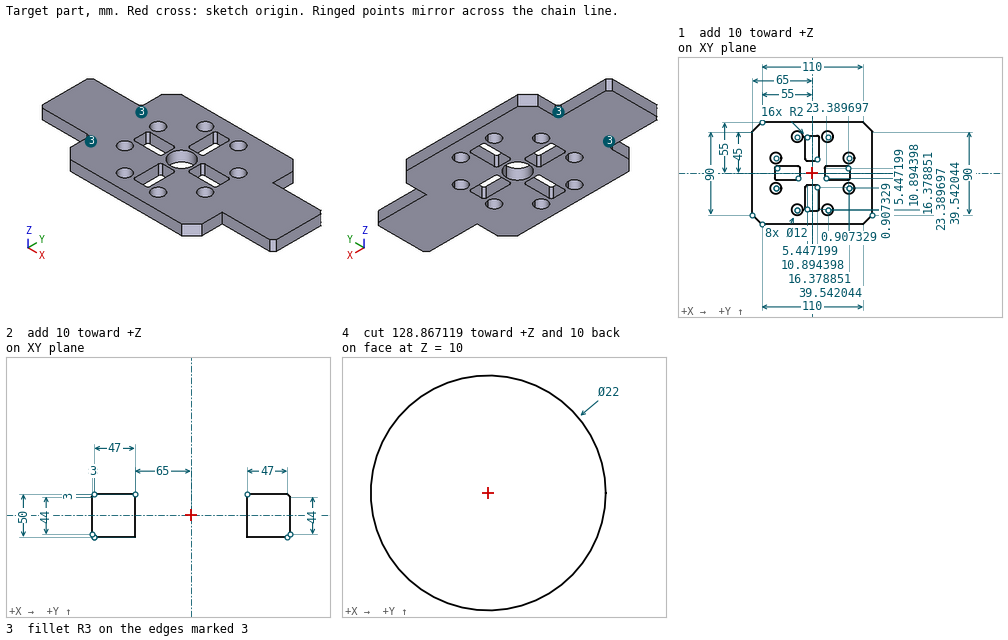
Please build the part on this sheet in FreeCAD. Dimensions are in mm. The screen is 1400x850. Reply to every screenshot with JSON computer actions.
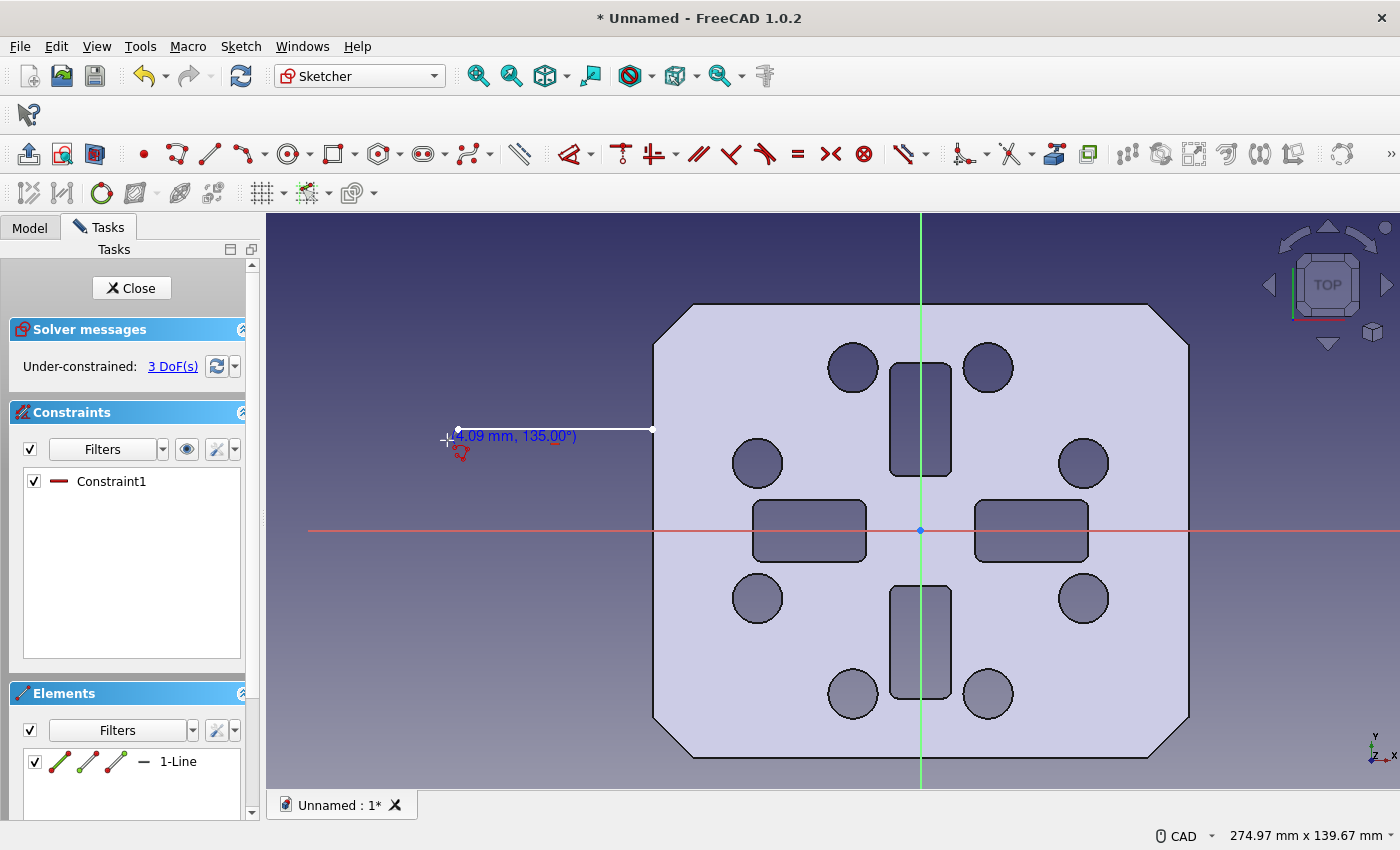
{"action": "left_click", "coordinate": [446, 440]}
{"action": "left_click", "coordinate": [446, 622]}
{"action": "left_click", "coordinate": [459, 634]}
{"action": "left_click", "coordinate": [653, 634]}
{"action": "left_click", "coordinate": [653, 429]}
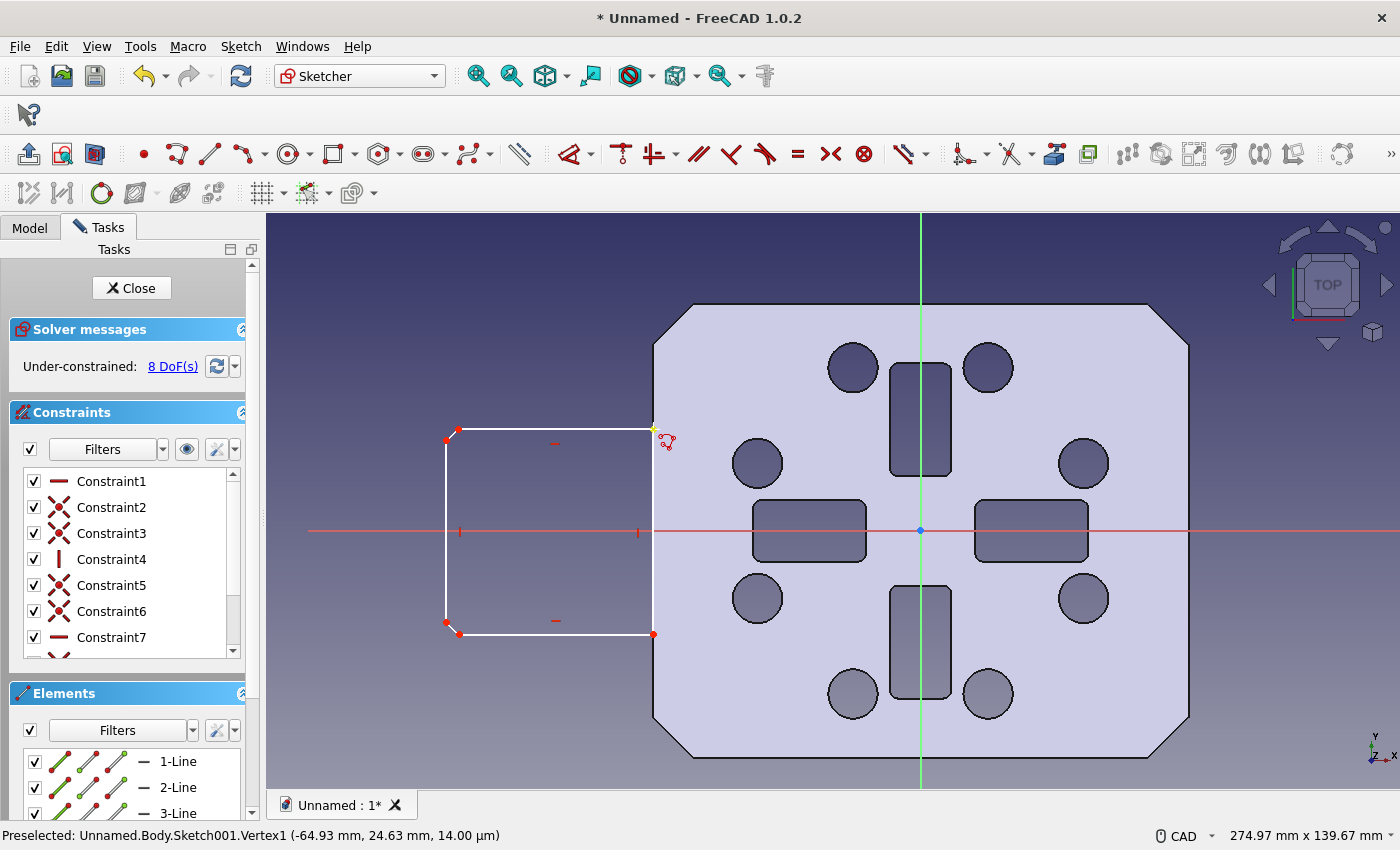
{"action": "left_click", "coordinate": [1189, 428]}
{"action": "left_click", "coordinate": [1189, 634]}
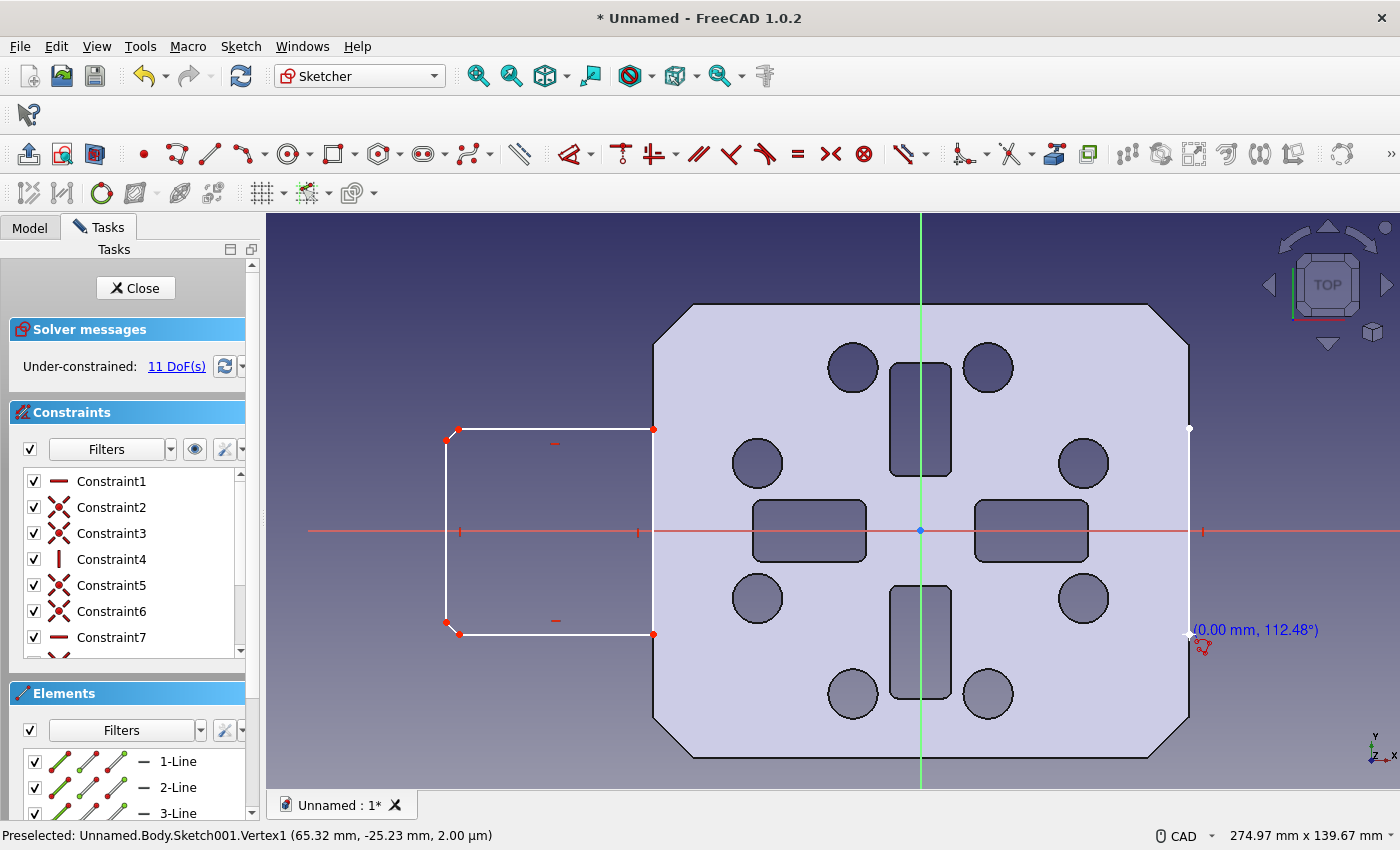
{"action": "scroll", "coordinate": [447, 440], "scroll_direction": "down", "scroll_amount": 2}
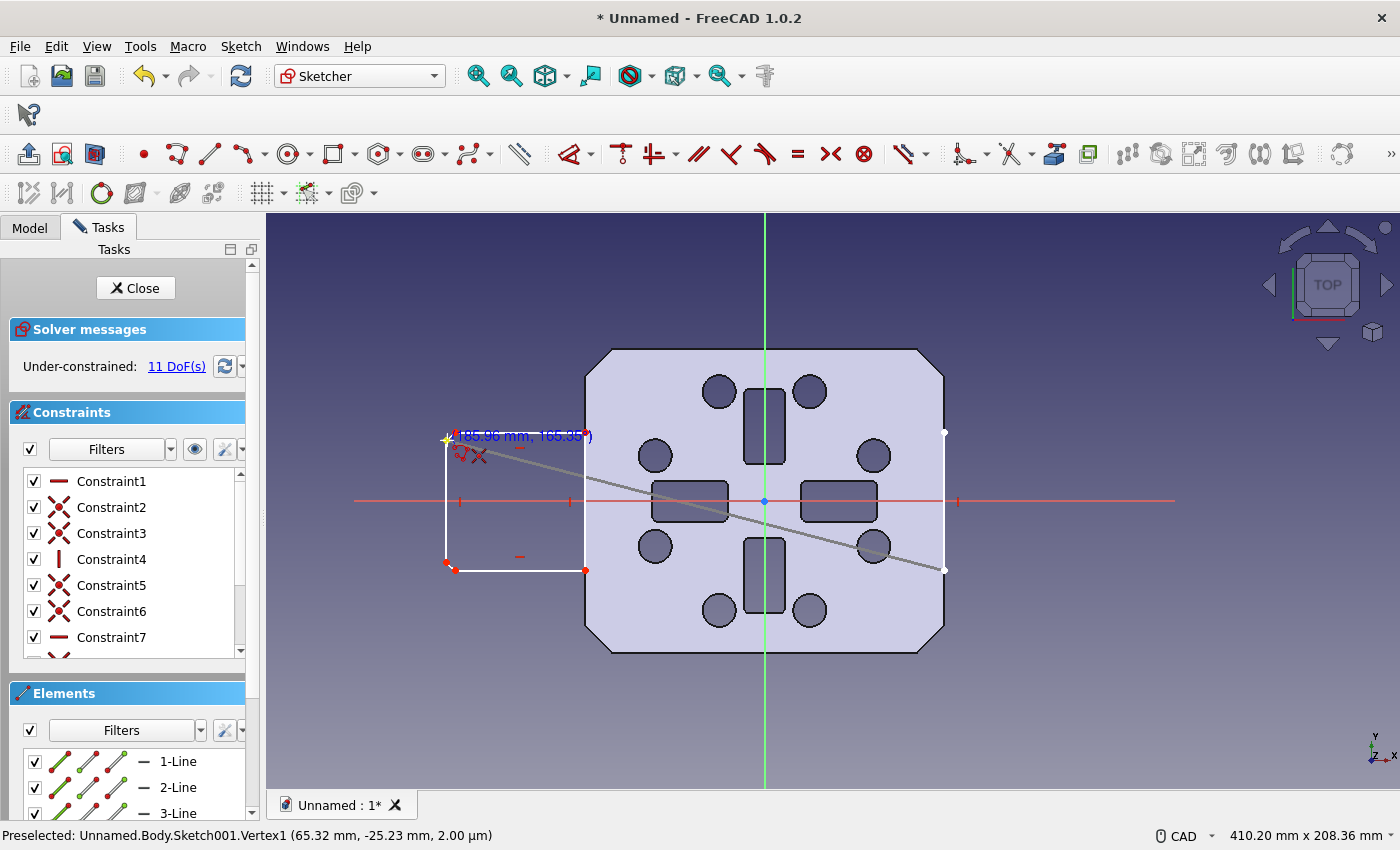
{"action": "left_click", "coordinate": [1074, 570]}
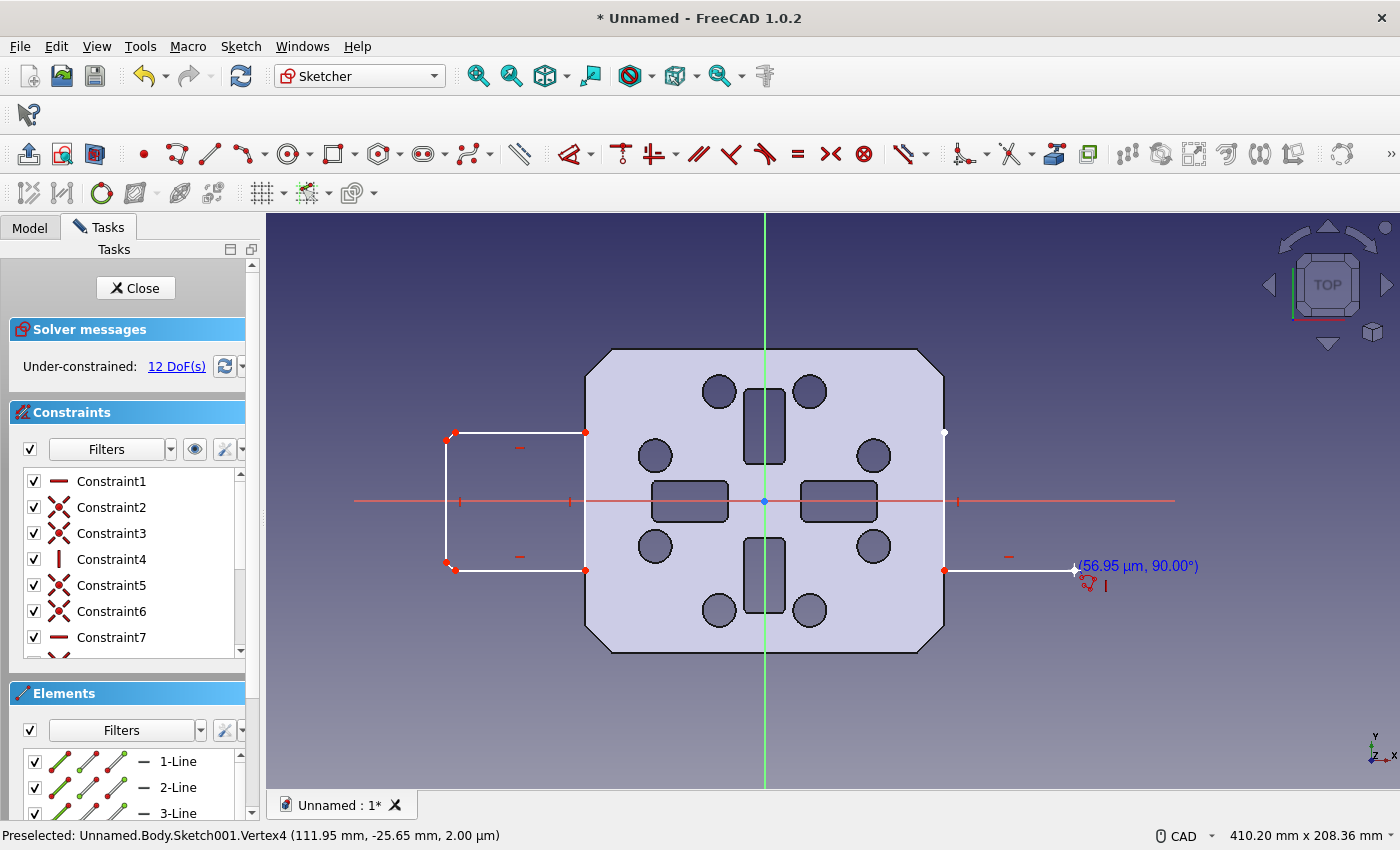
{"action": "scroll", "coordinate": [1082, 562], "scroll_direction": "up", "scroll_amount": 2}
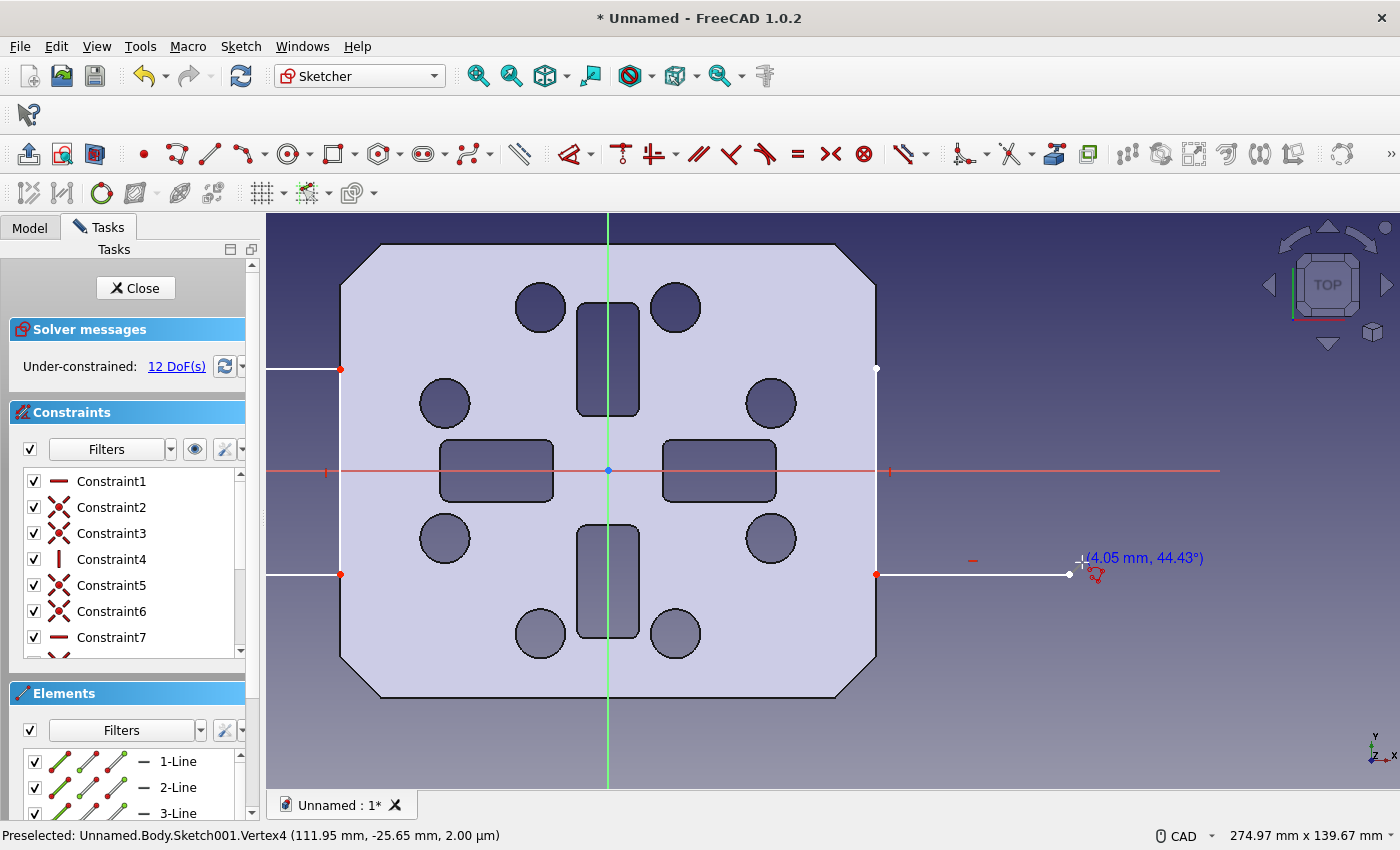
{"action": "left_click", "coordinate": [1082, 562]}
{"action": "left_click", "coordinate": [1082, 380]}
{"action": "left_click", "coordinate": [1070, 368]}
{"action": "left_click", "coordinate": [876, 369]}
{"action": "key", "text": "Escape"}
{"action": "key", "text": "Escape"}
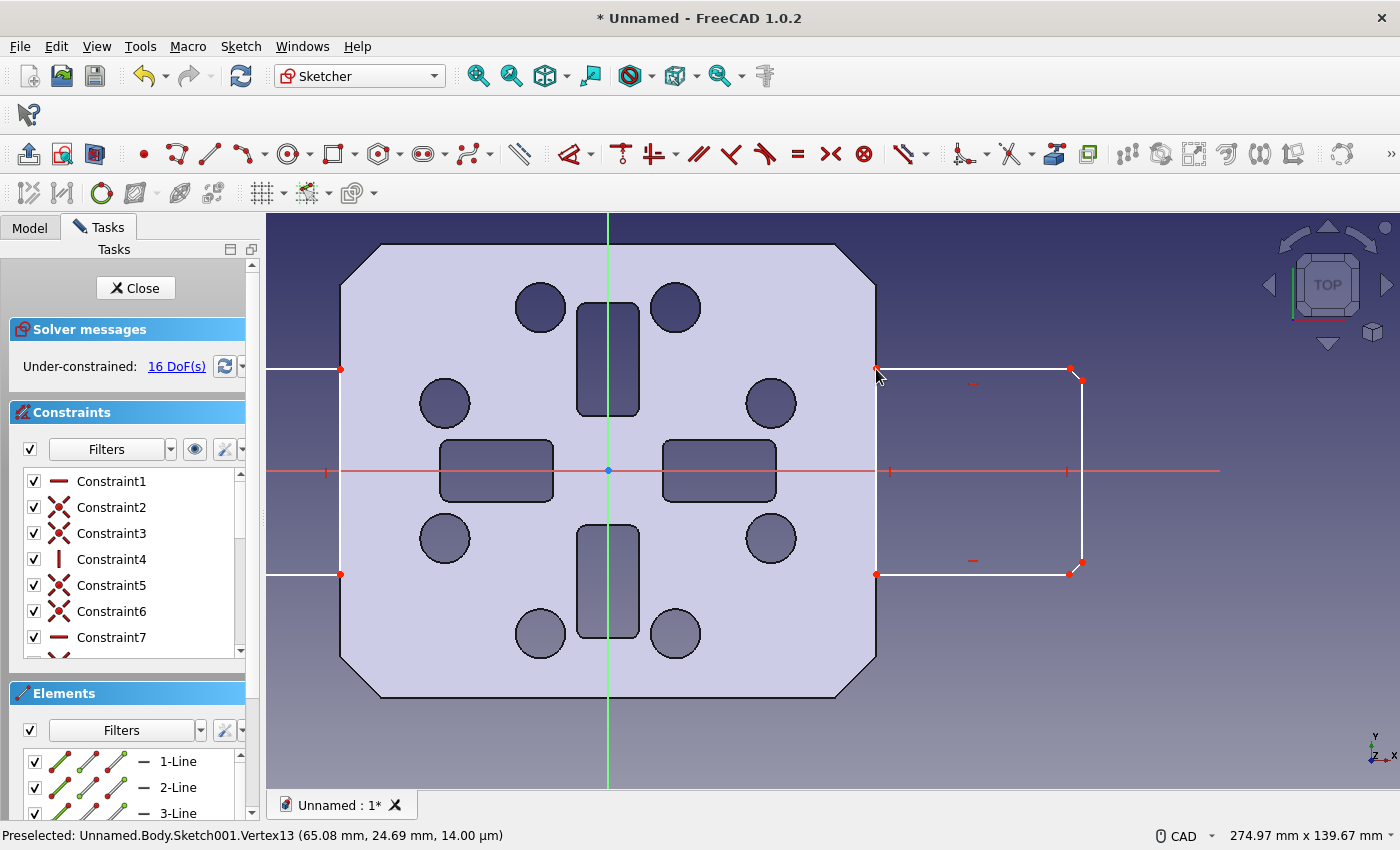
{"action": "scroll", "coordinate": [1083, 562], "scroll_direction": "down", "scroll_amount": 2}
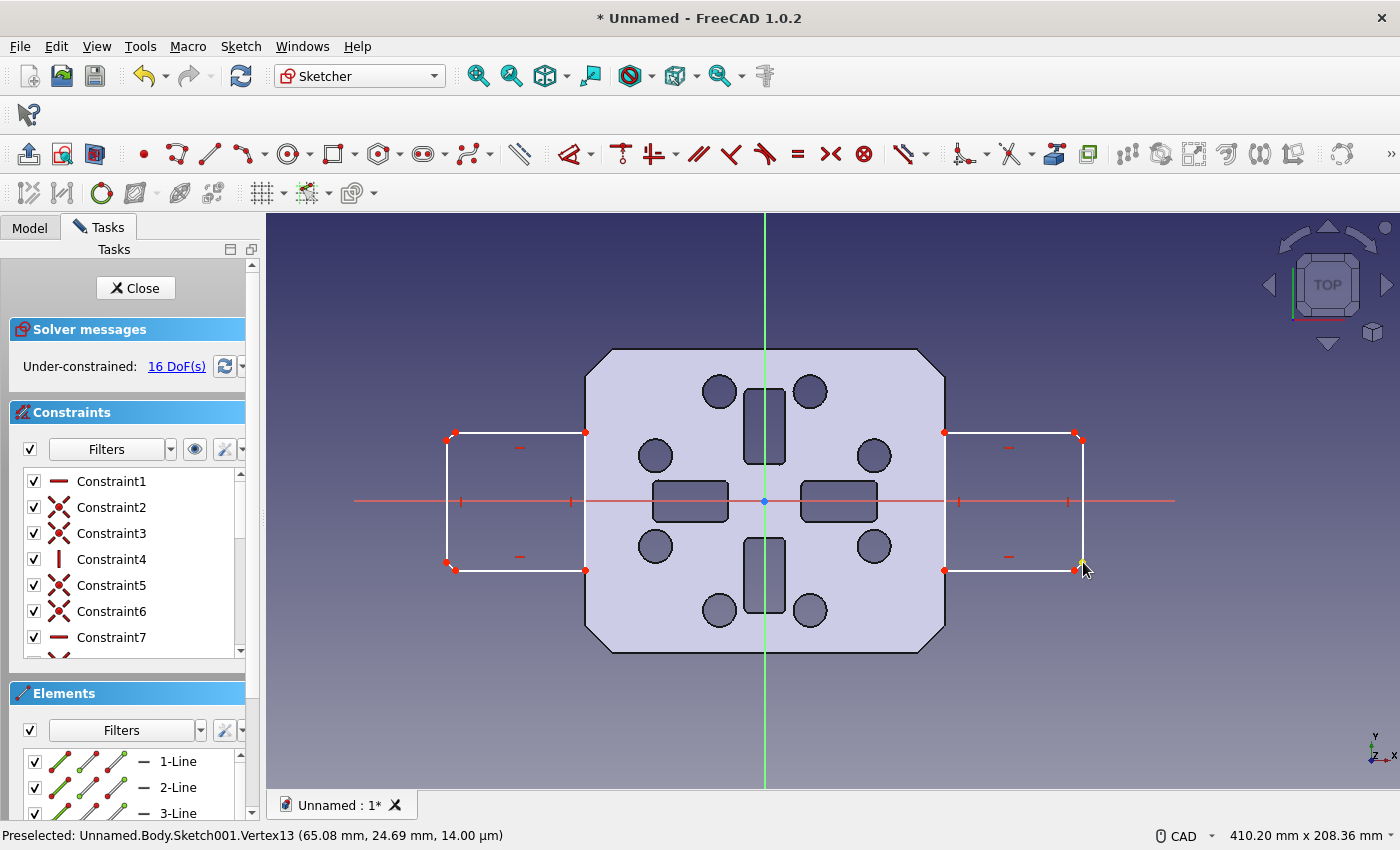
{"action": "left_click", "coordinate": [455, 433]}